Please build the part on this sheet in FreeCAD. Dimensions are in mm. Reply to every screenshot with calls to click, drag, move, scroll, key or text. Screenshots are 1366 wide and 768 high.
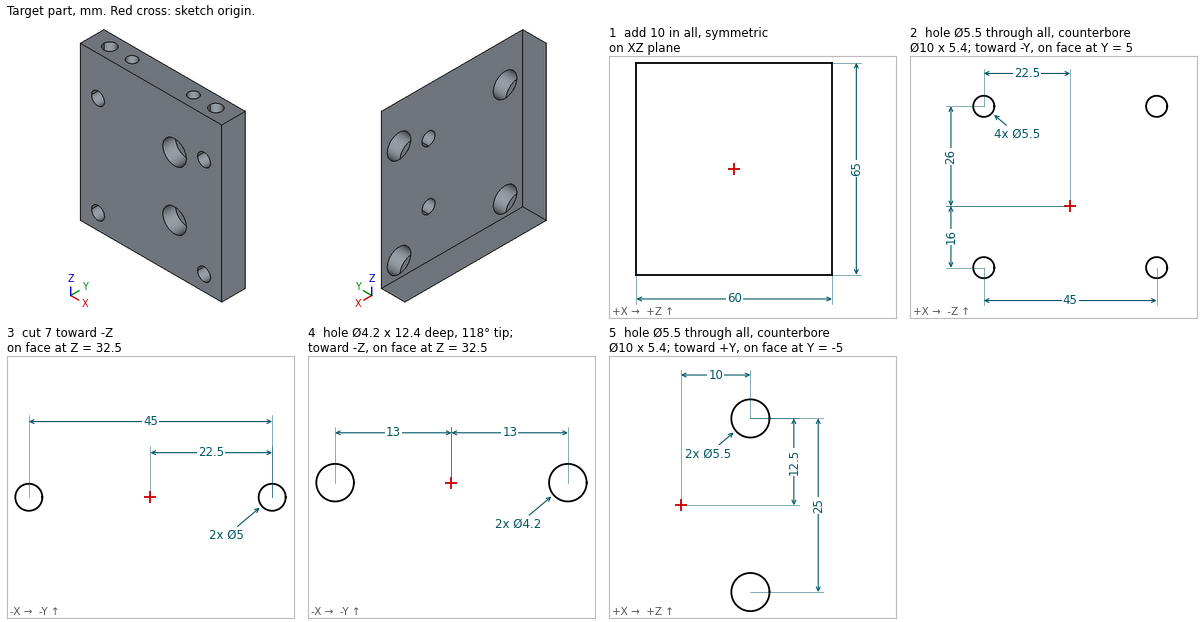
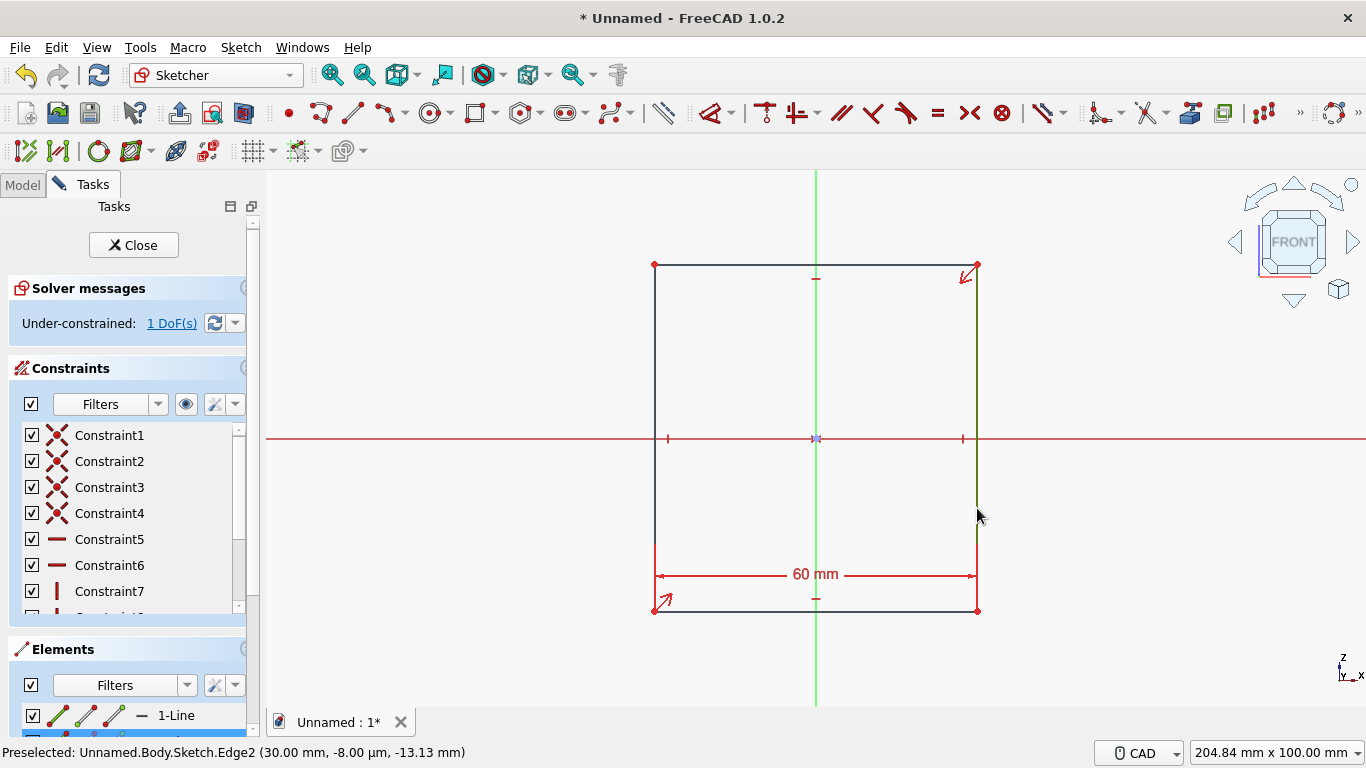
key(i)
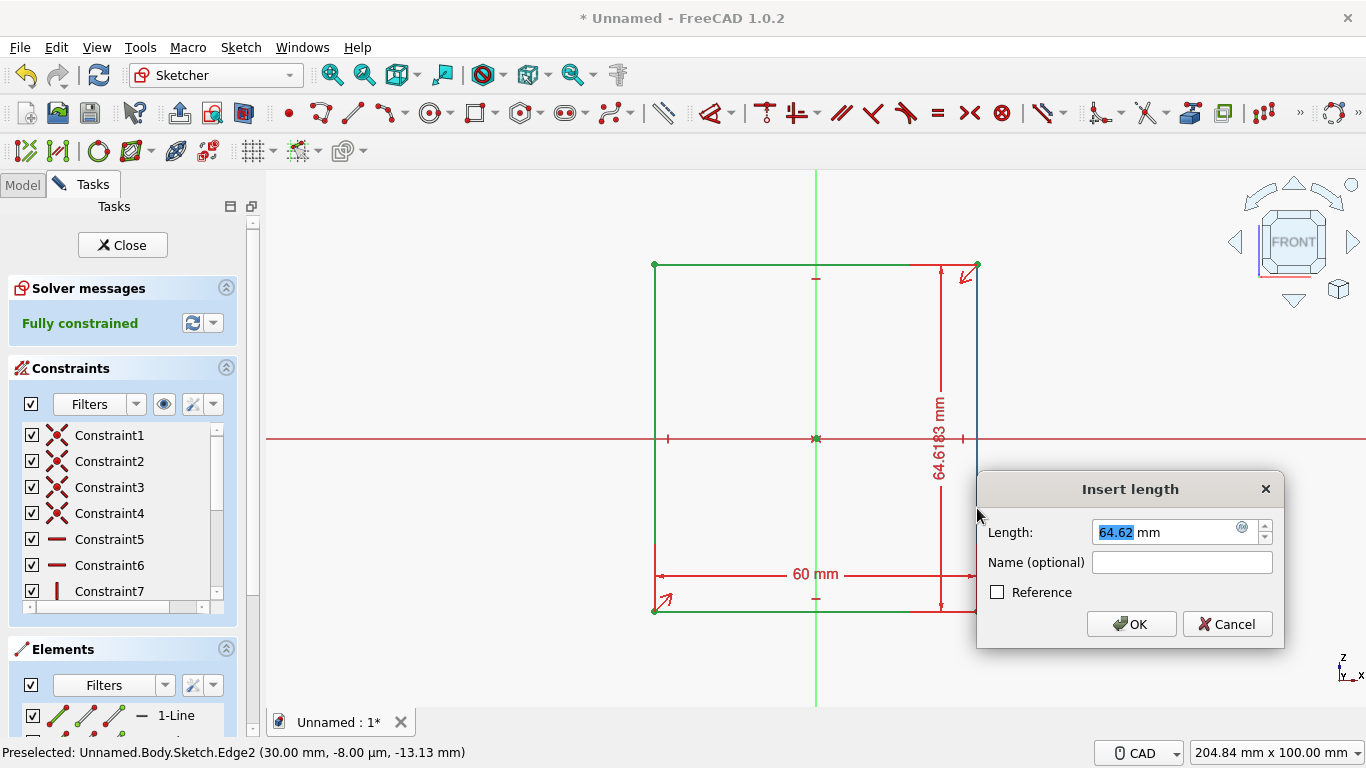
text(65)
key(Return)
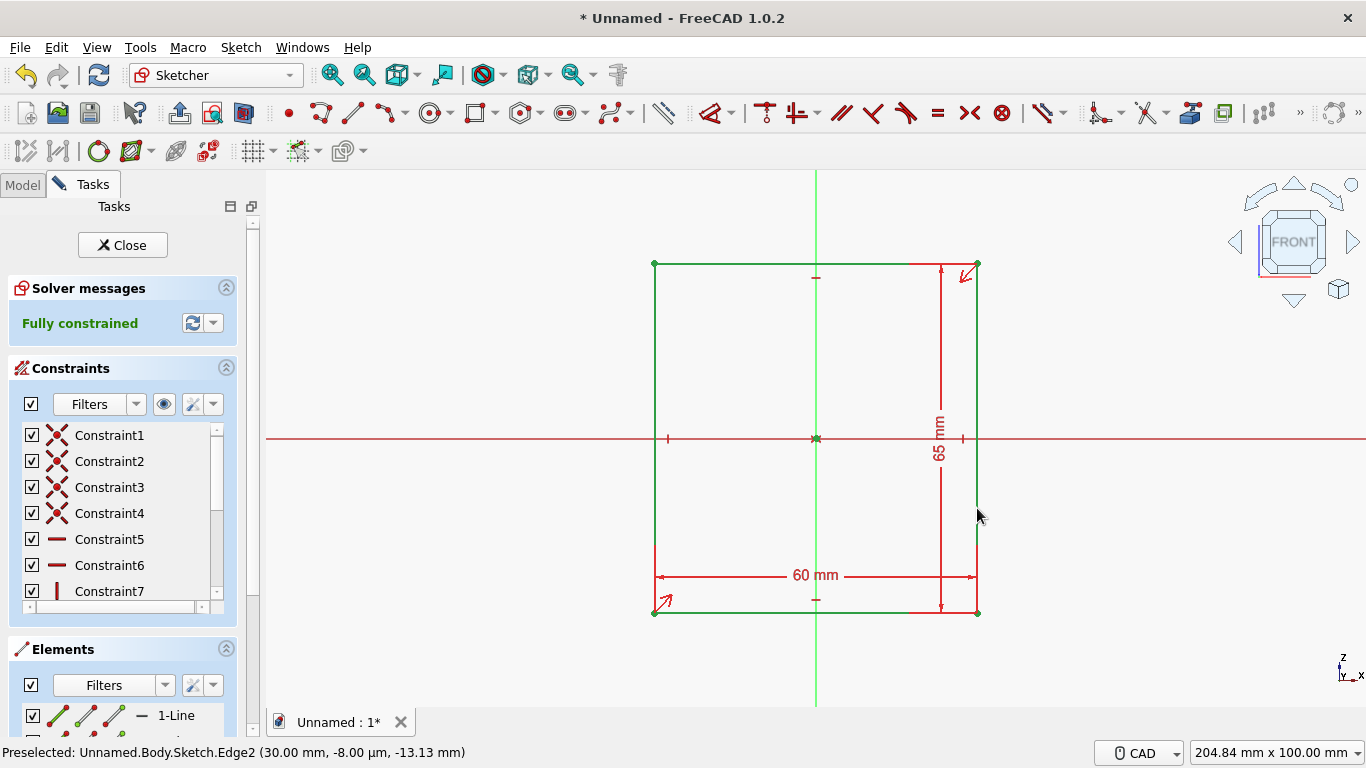
click(123, 245)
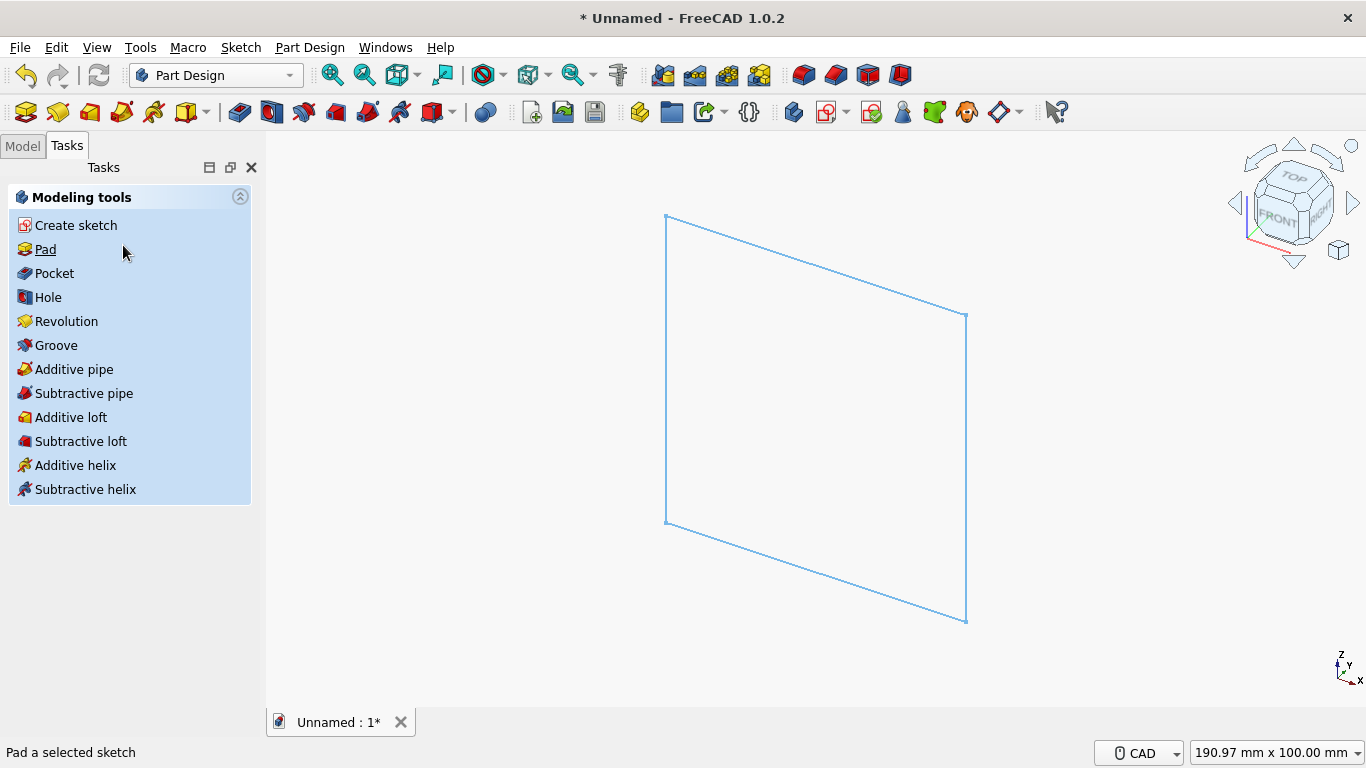
click(26, 112)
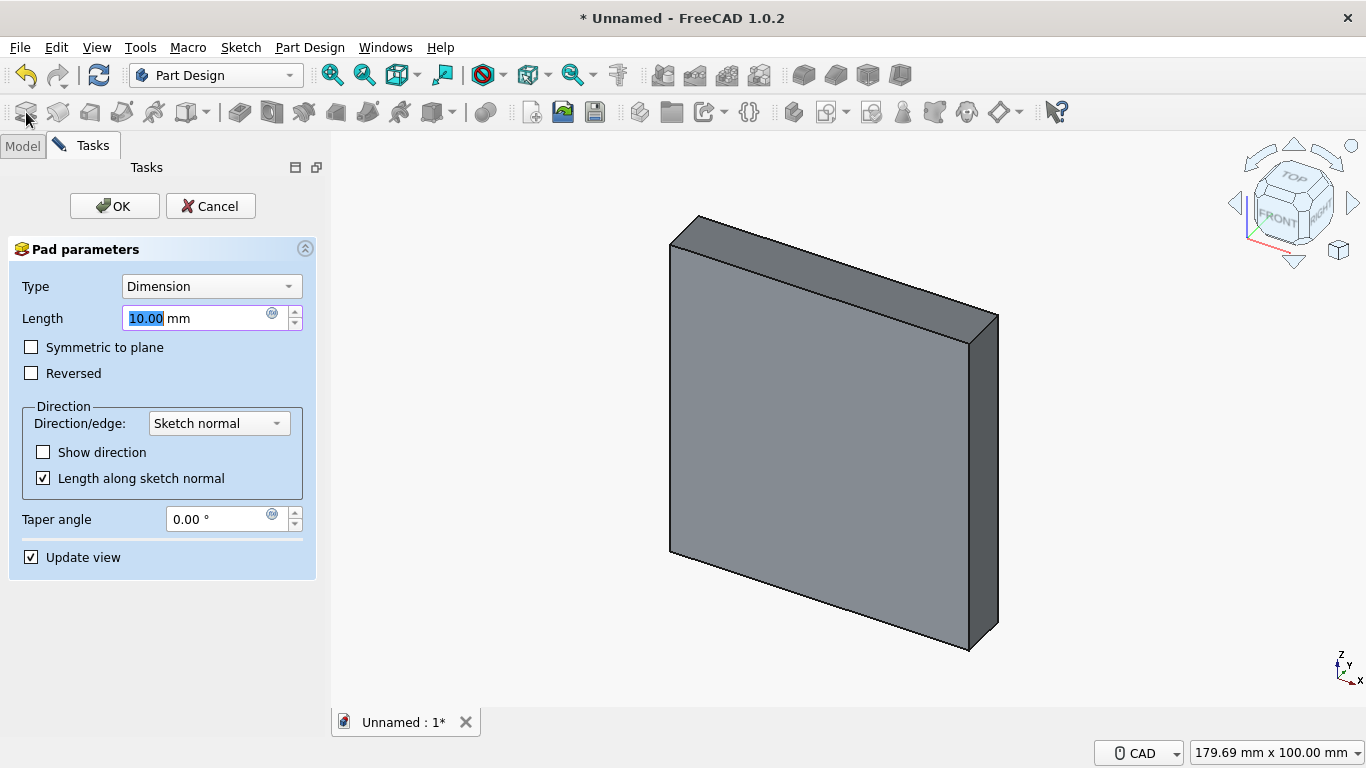
text(10)
key(Tab)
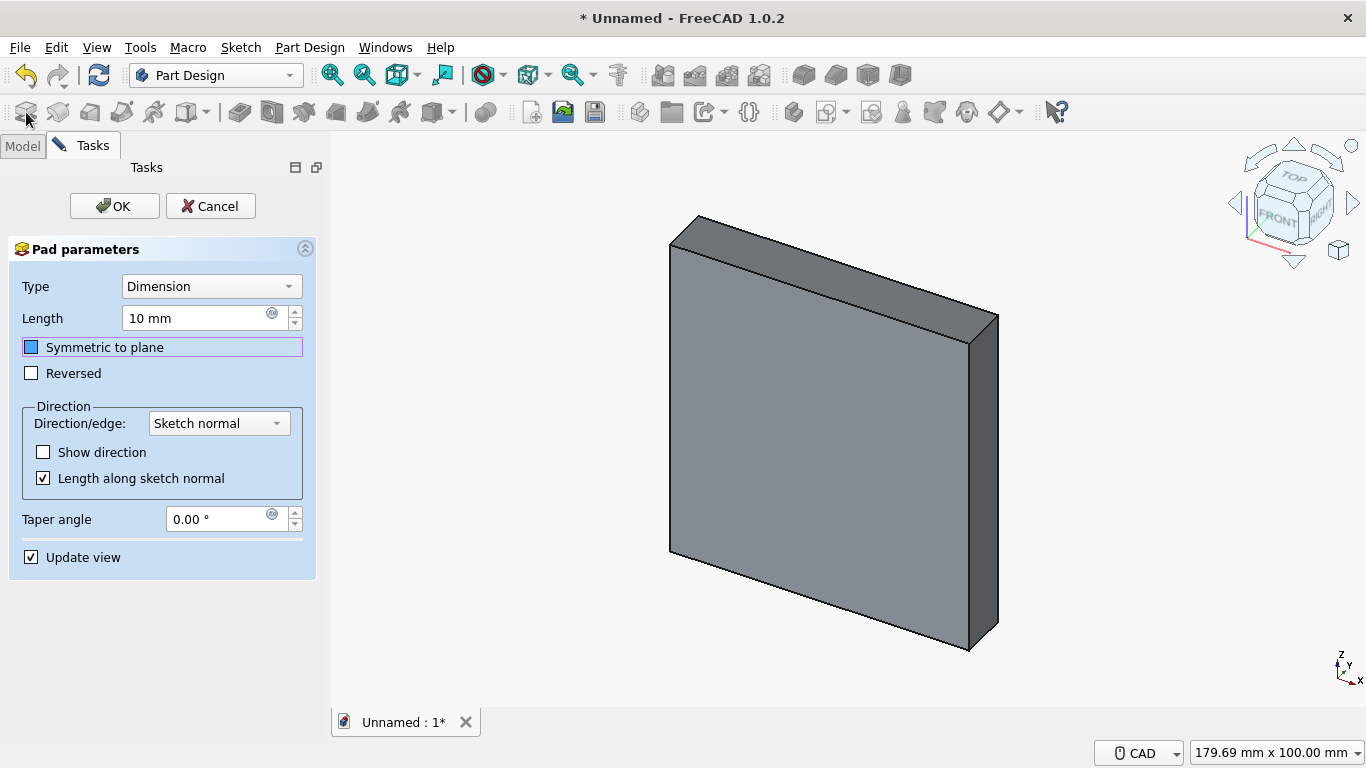
click(30, 347)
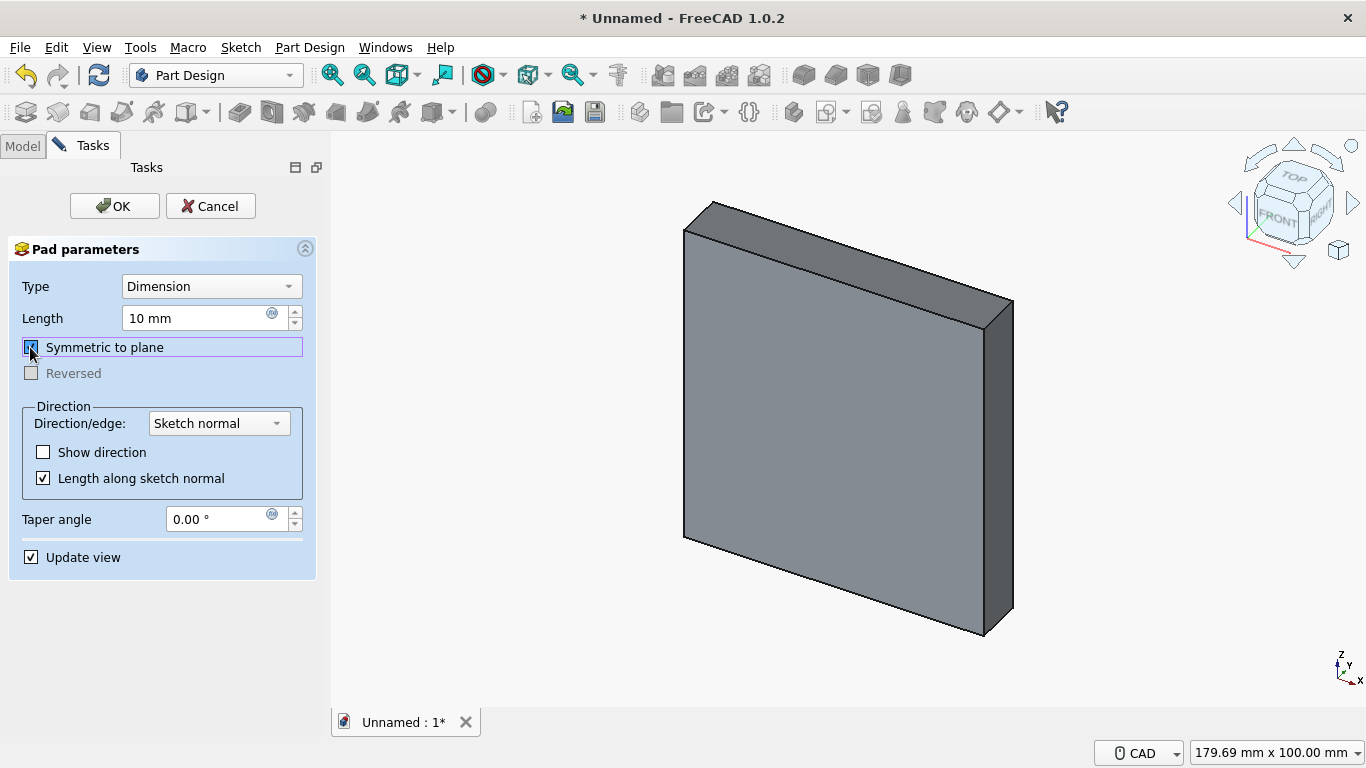
click(115, 206)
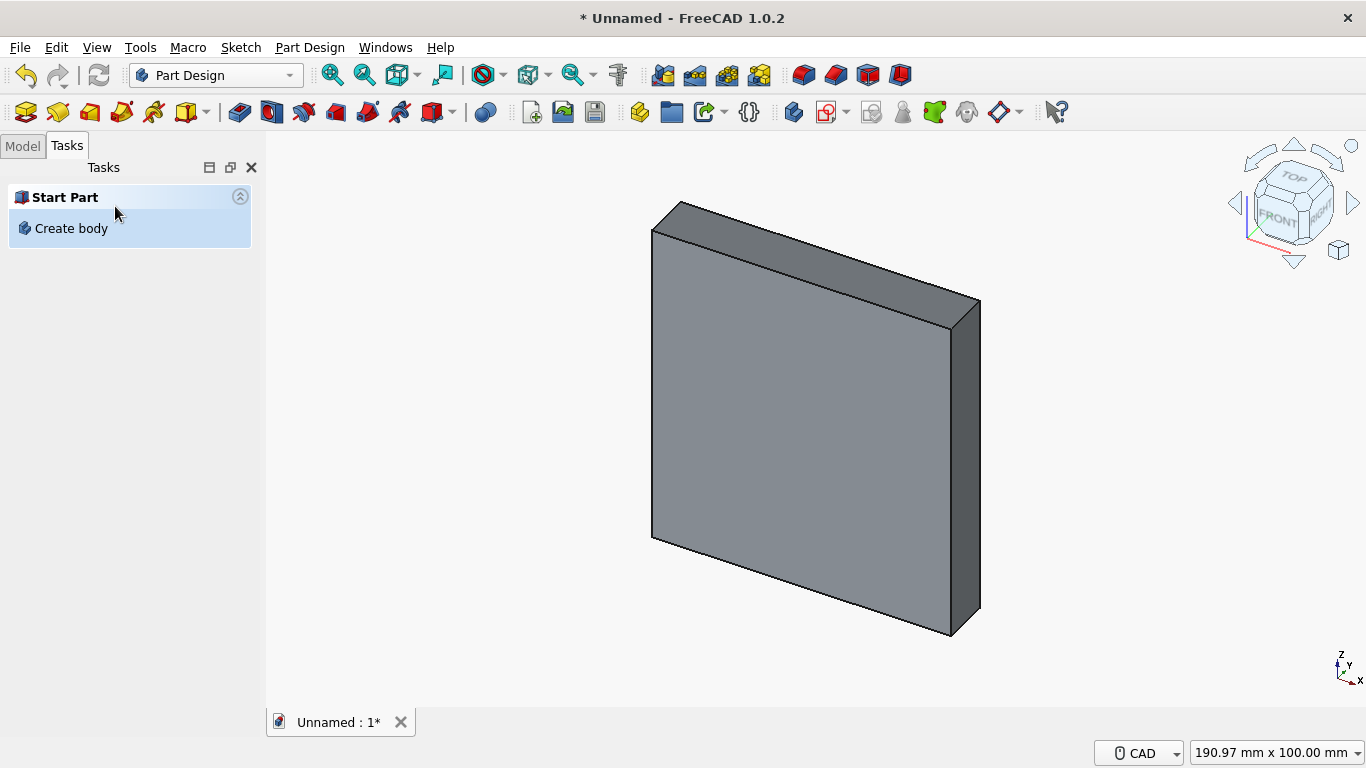
key(4)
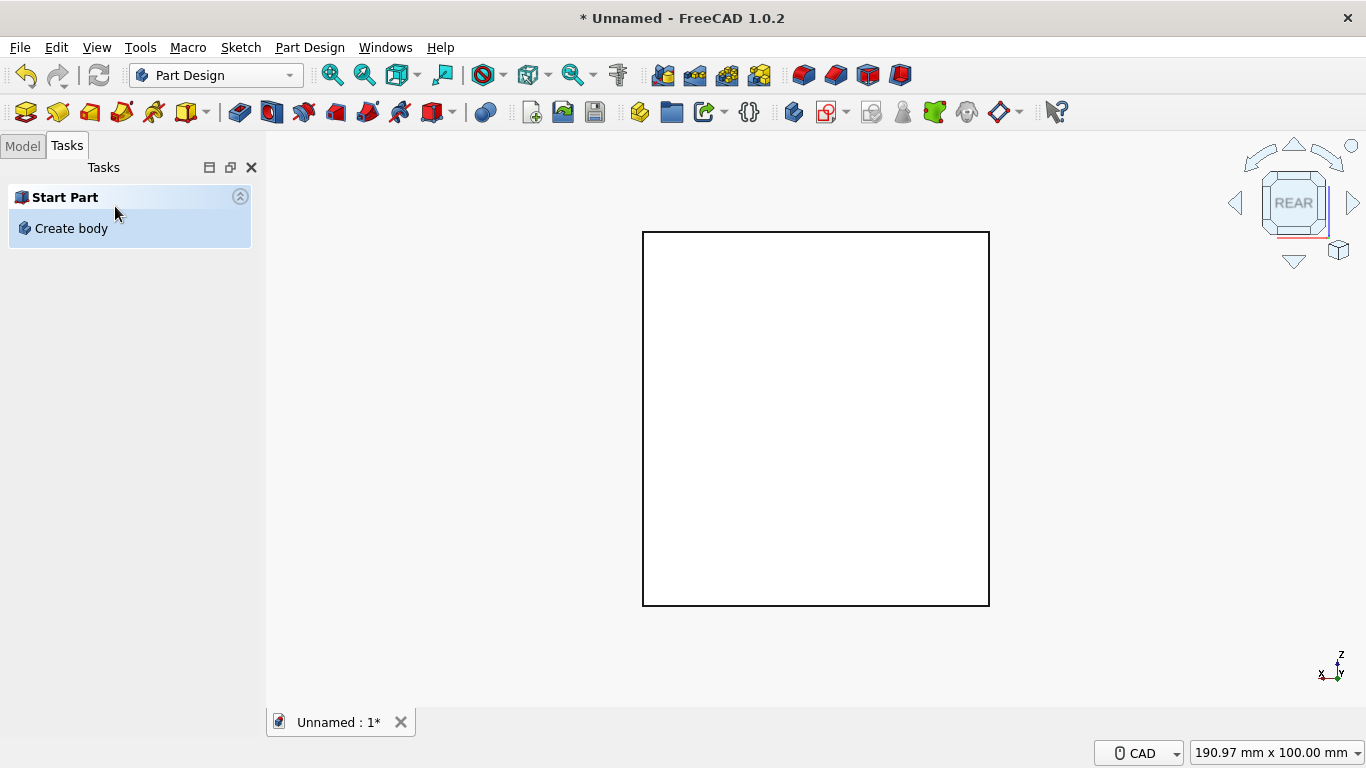
click(816, 418)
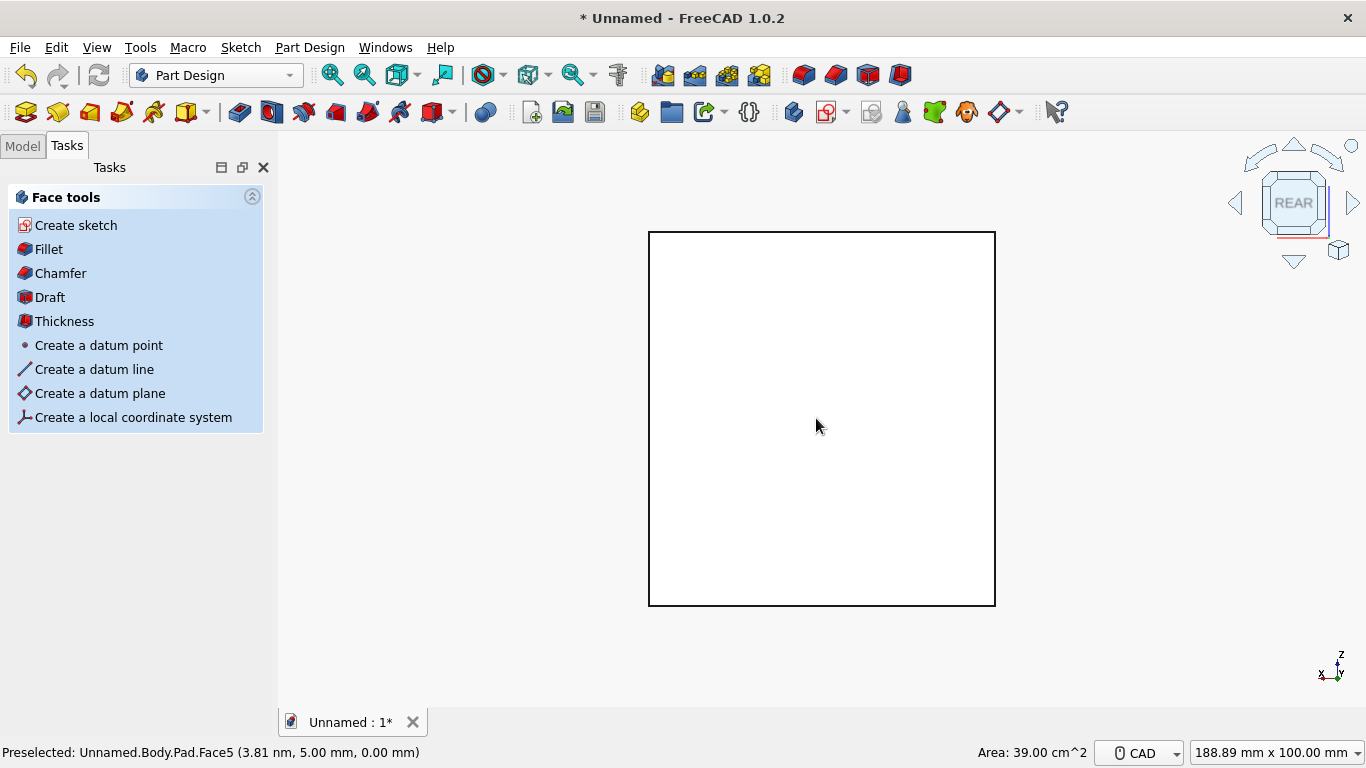
click(826, 112)